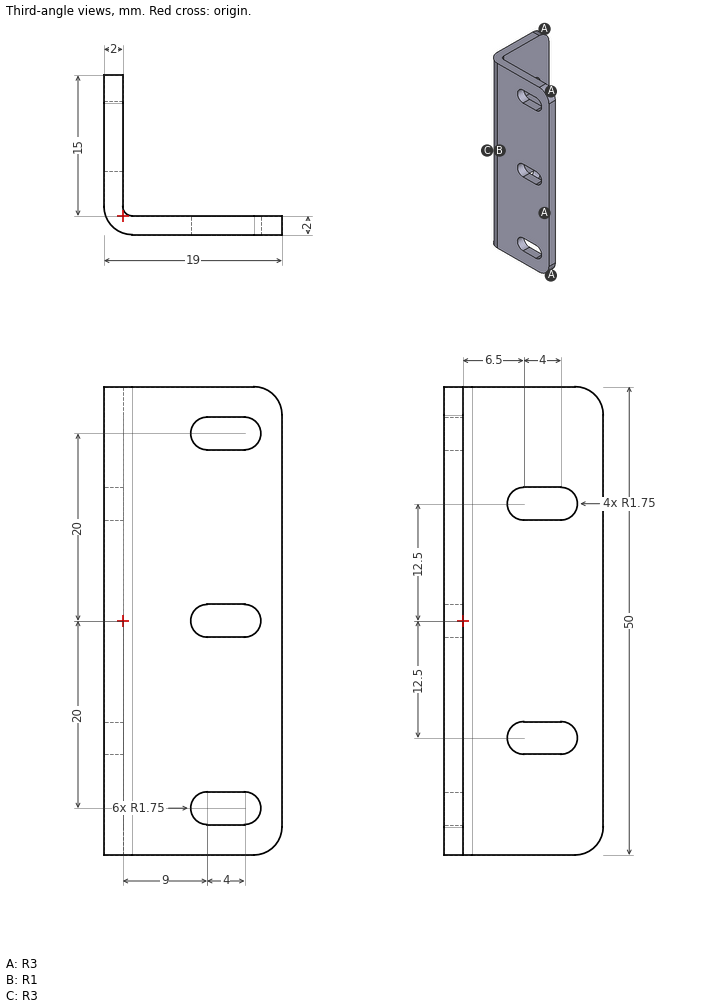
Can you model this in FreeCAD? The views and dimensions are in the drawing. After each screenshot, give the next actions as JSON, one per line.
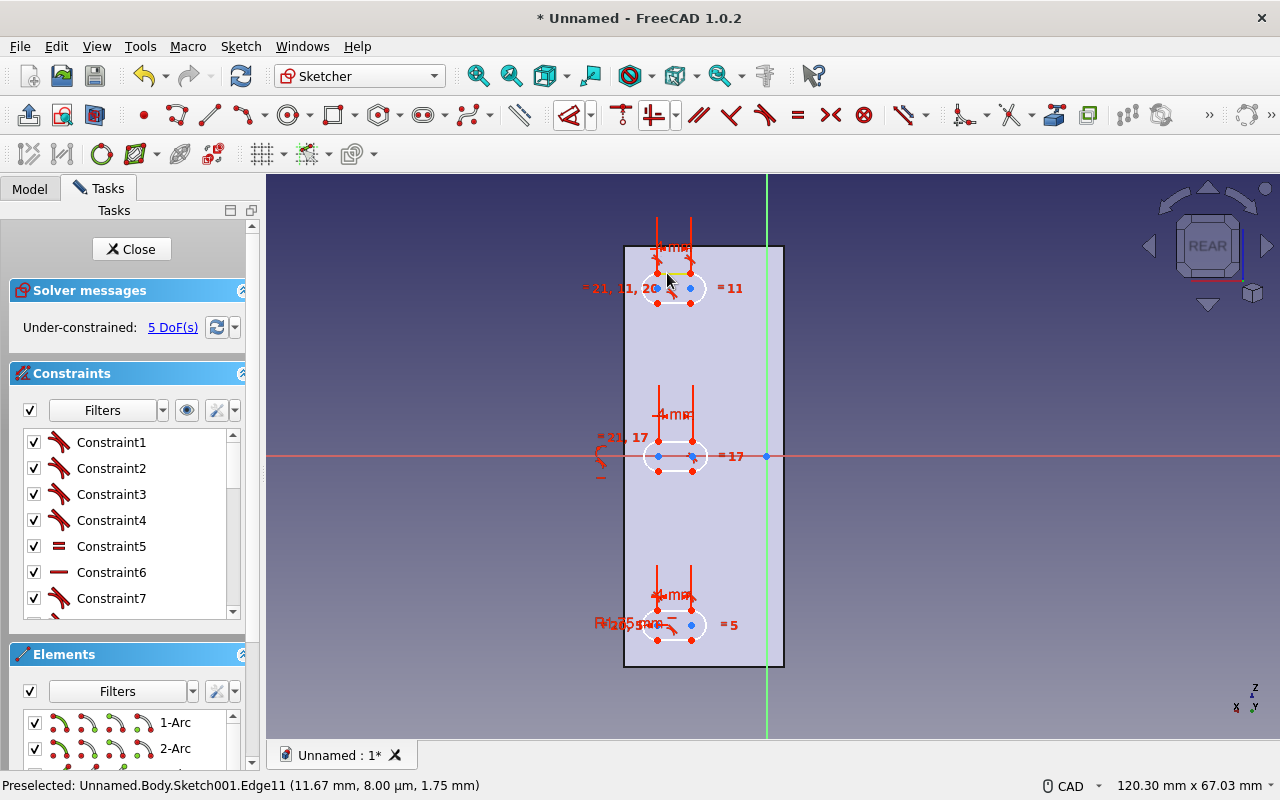
{"action": "left_click", "coordinate": [691, 640]}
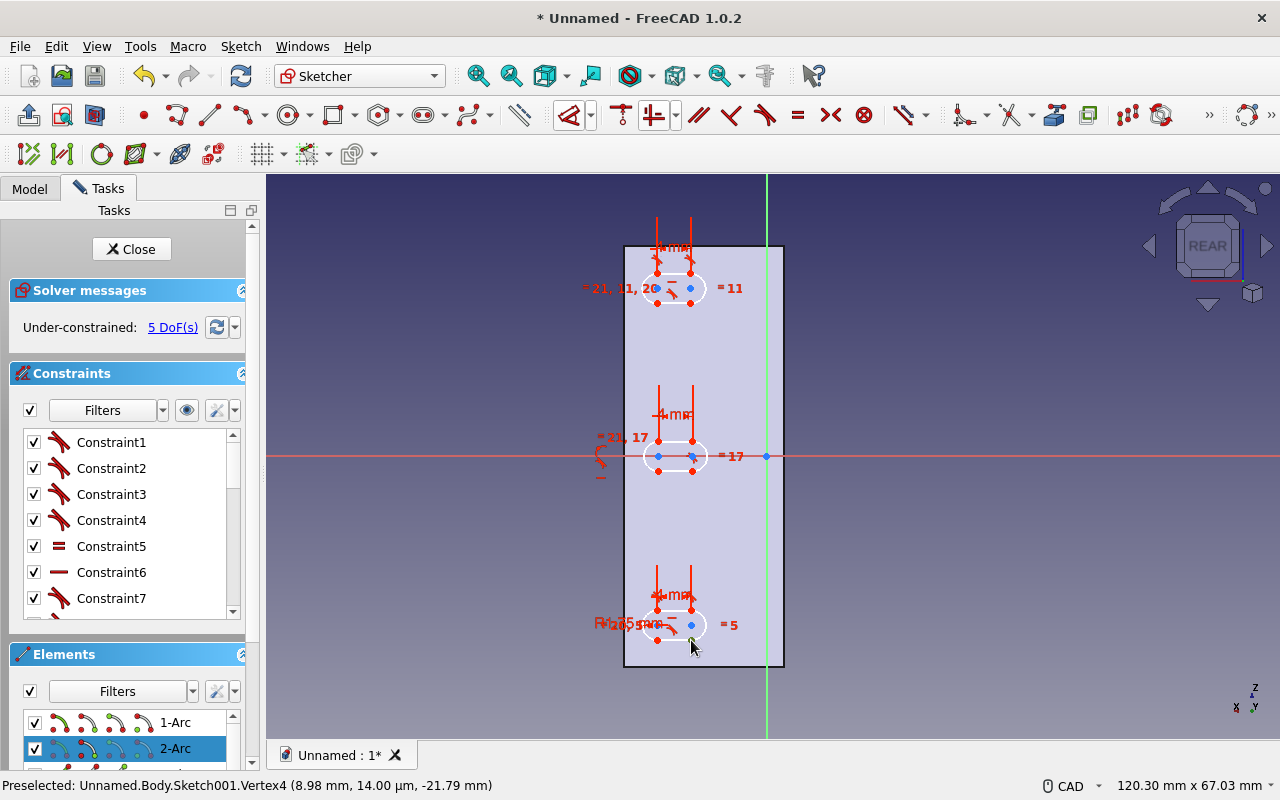
{"action": "key", "text": "l"}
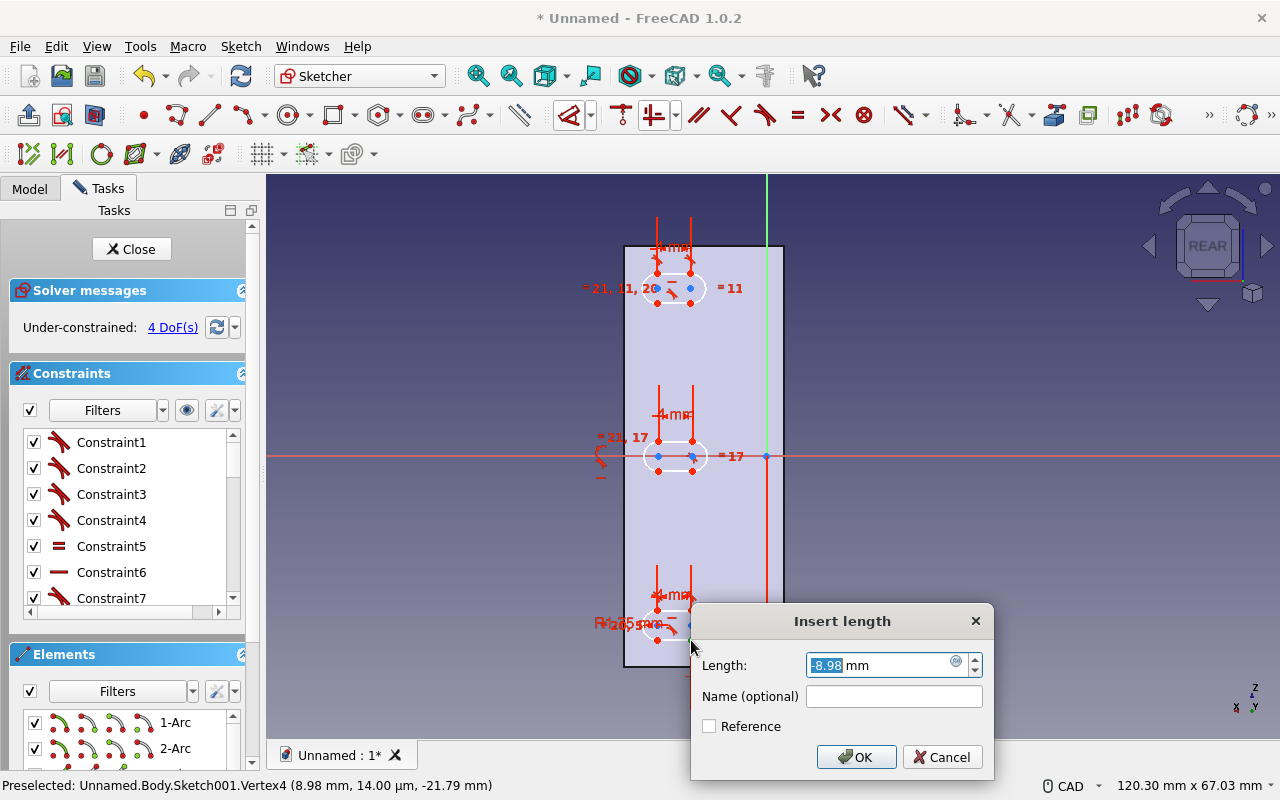
{"action": "type", "text": "-9"}
{"action": "key", "text": "Return"}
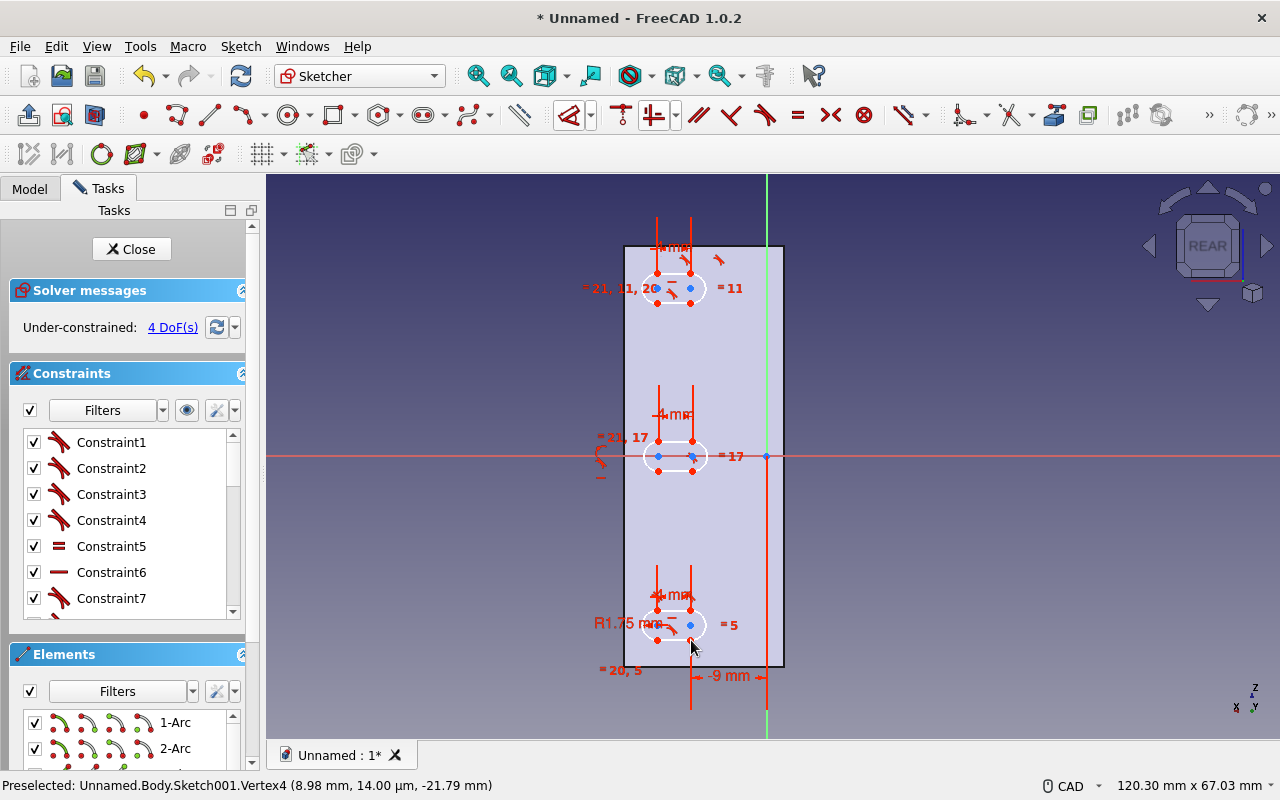
{"action": "left_click", "coordinate": [691, 303]}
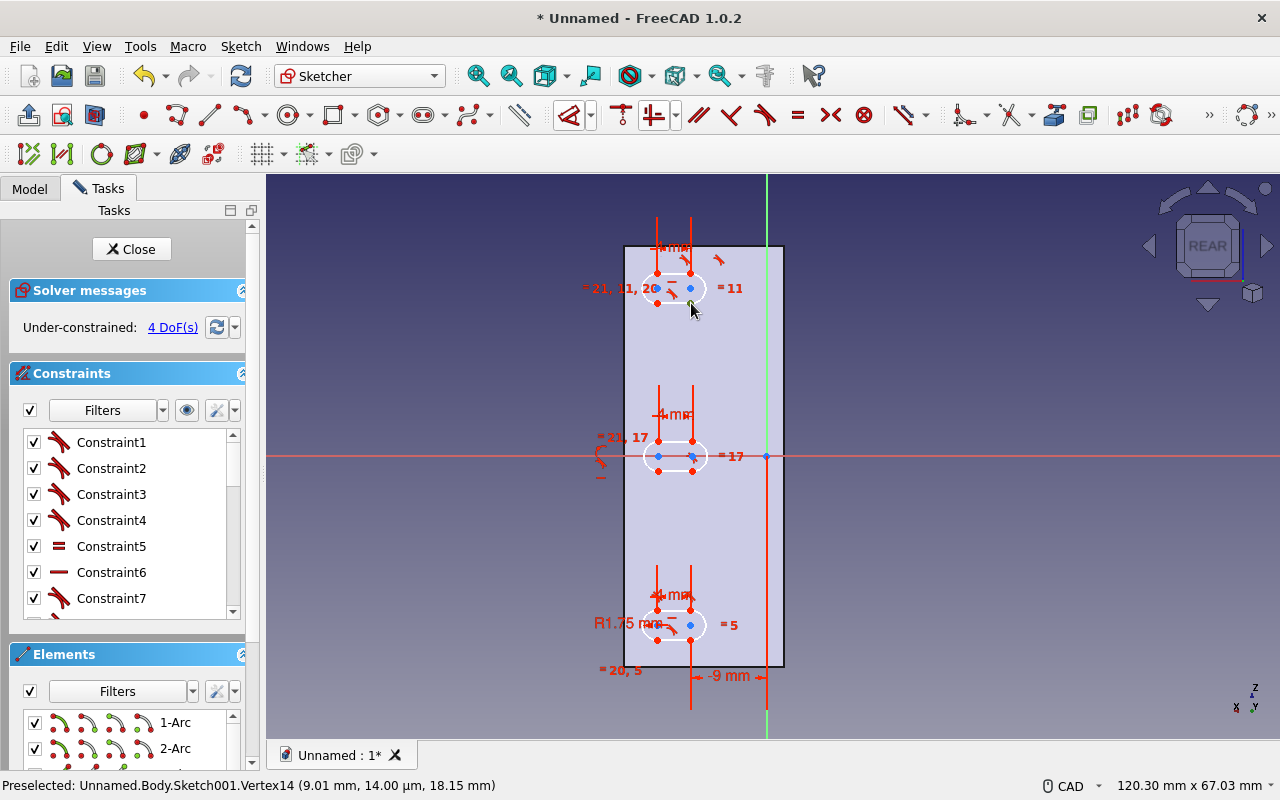
{"action": "key", "text": "l"}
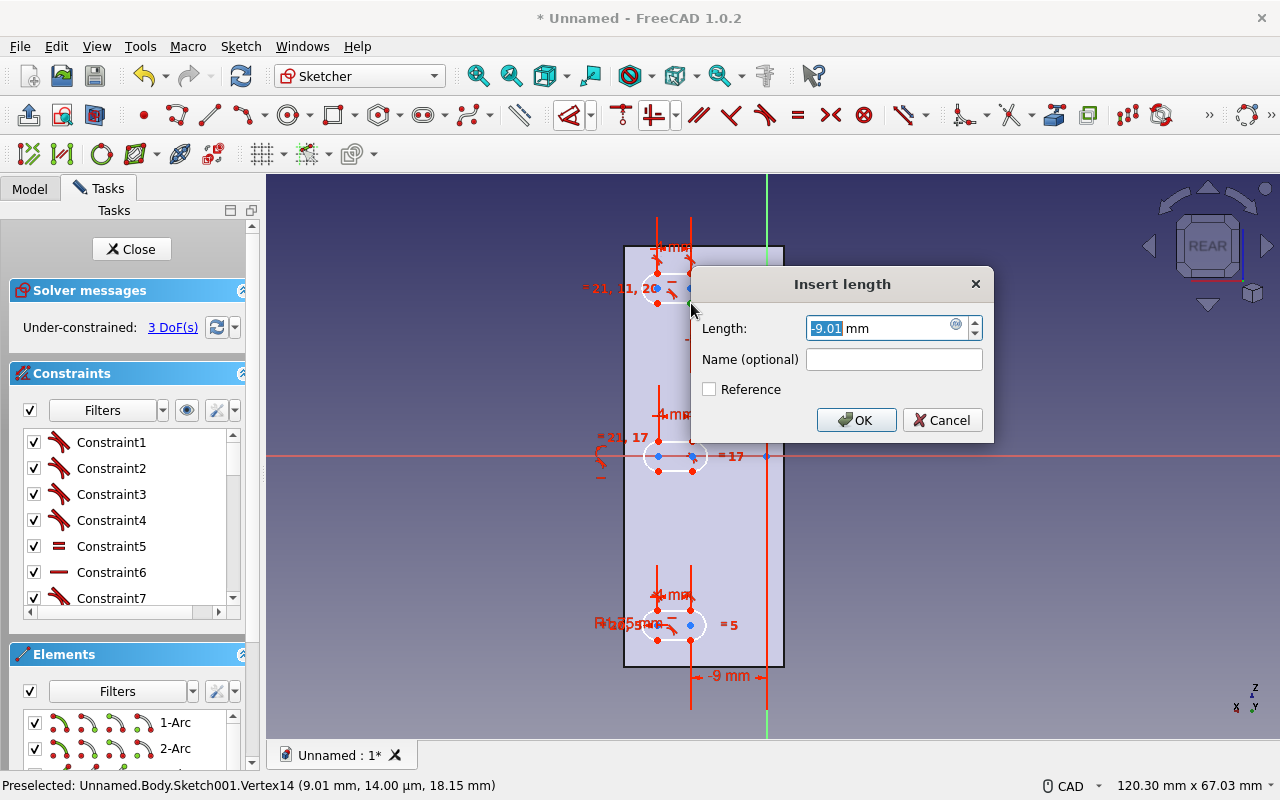
{"action": "type", "text": "-9"}
{"action": "key", "text": "Return"}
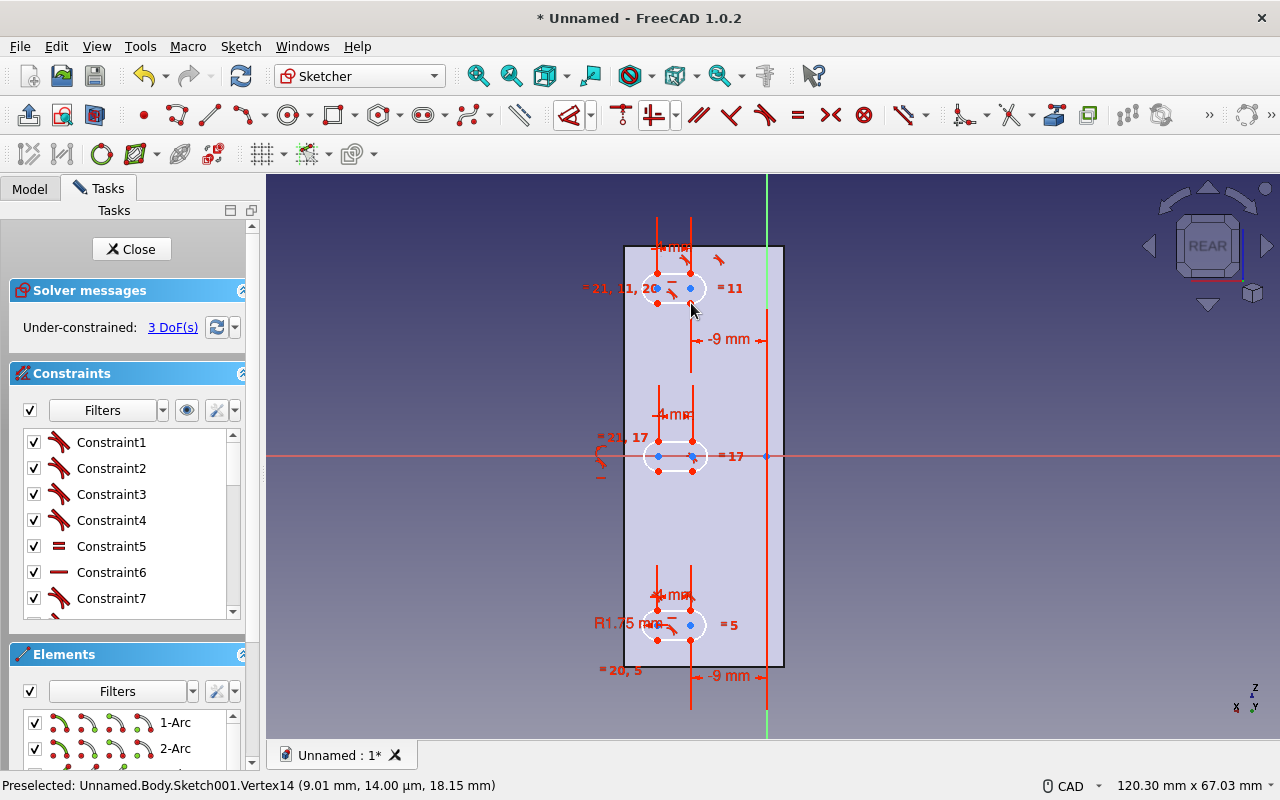
{"action": "left_click", "coordinate": [693, 471]}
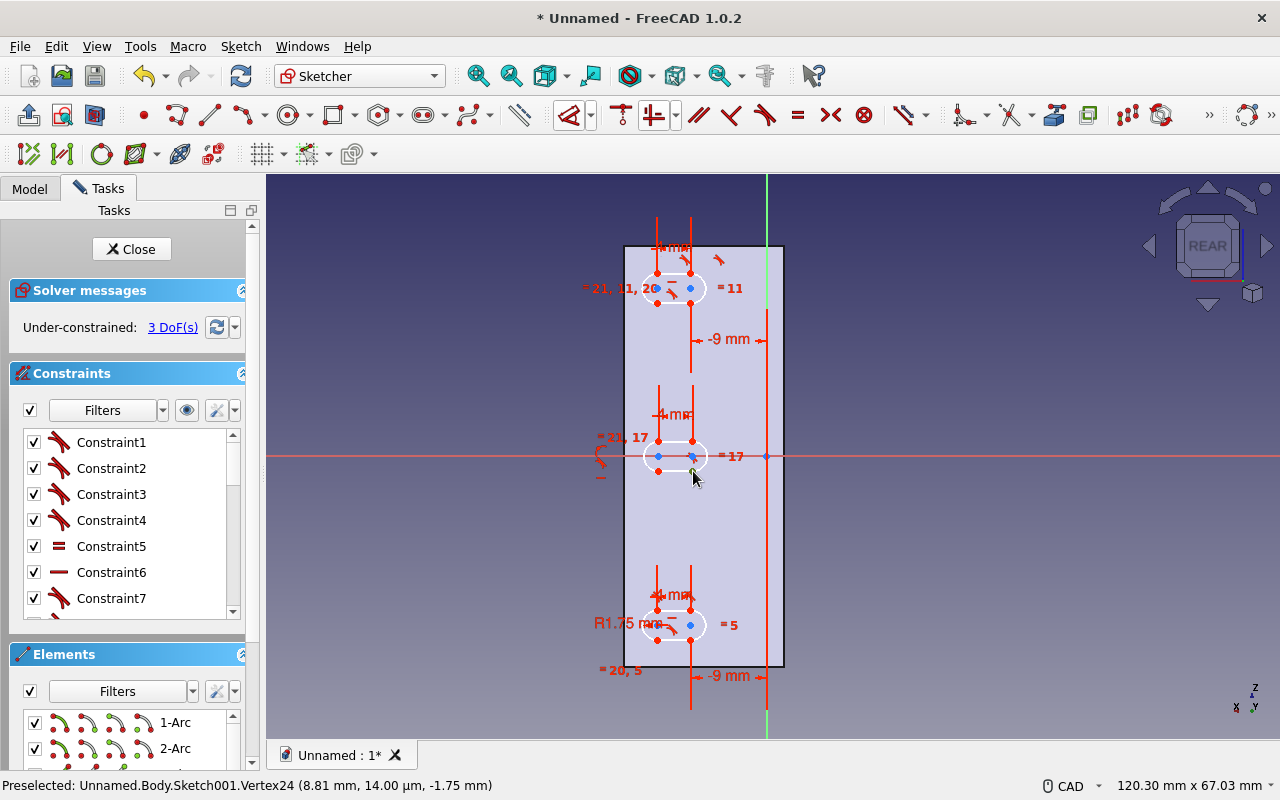
{"action": "key", "text": "l"}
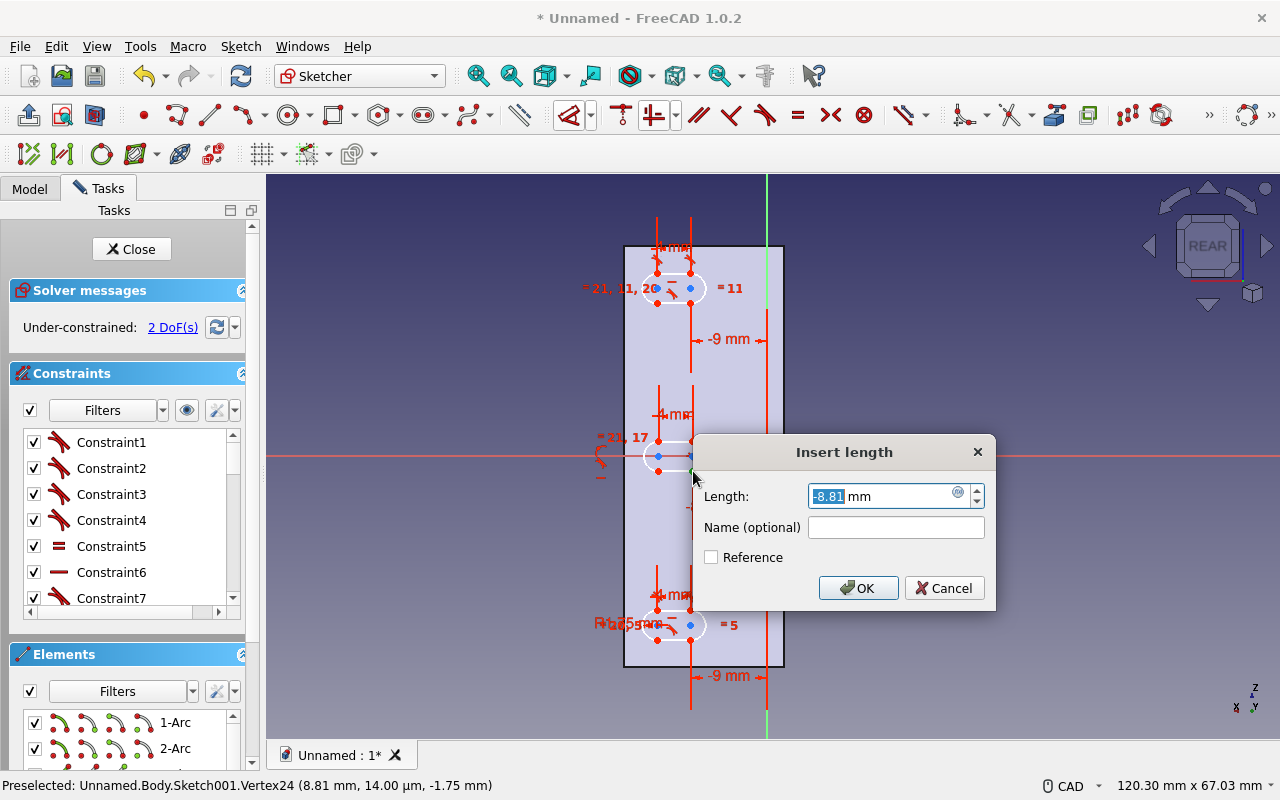
{"action": "type", "text": "-9"}
{"action": "key", "text": "Return"}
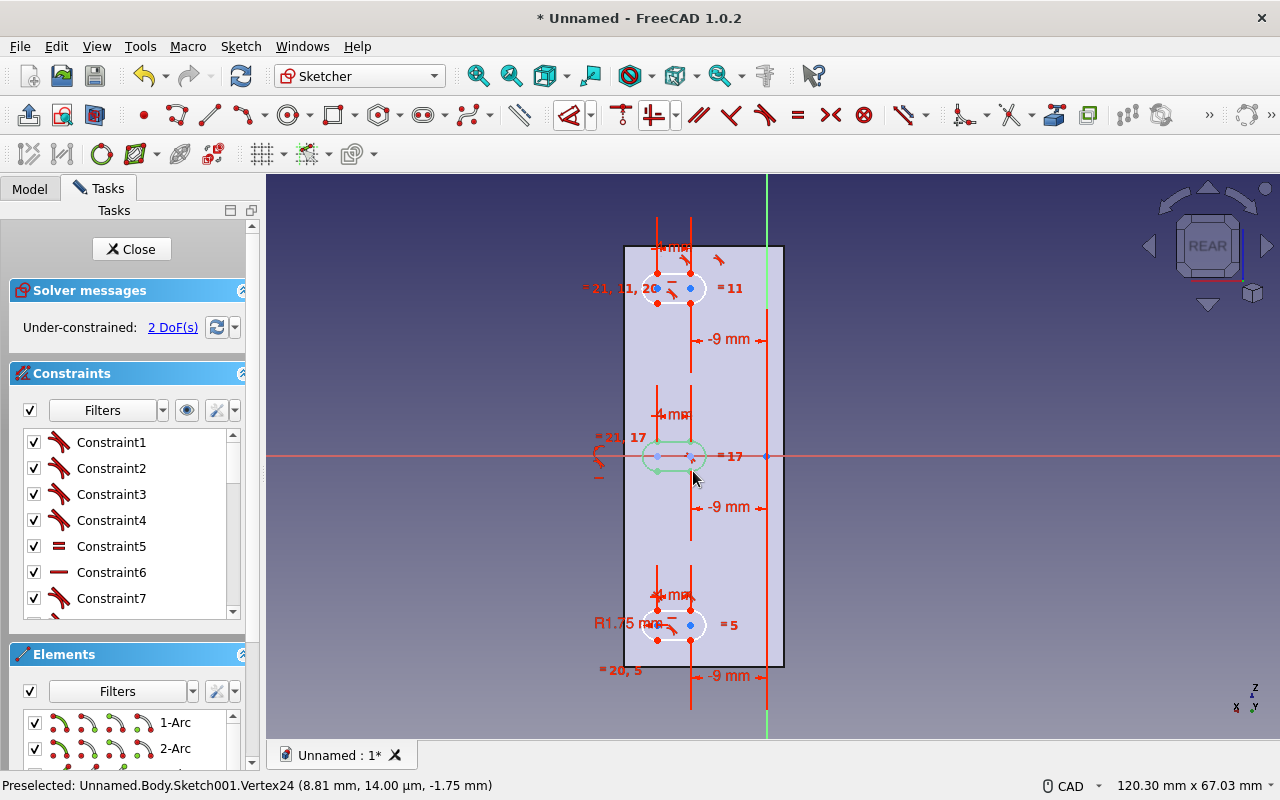
{"action": "left_click", "coordinate": [657, 625]}